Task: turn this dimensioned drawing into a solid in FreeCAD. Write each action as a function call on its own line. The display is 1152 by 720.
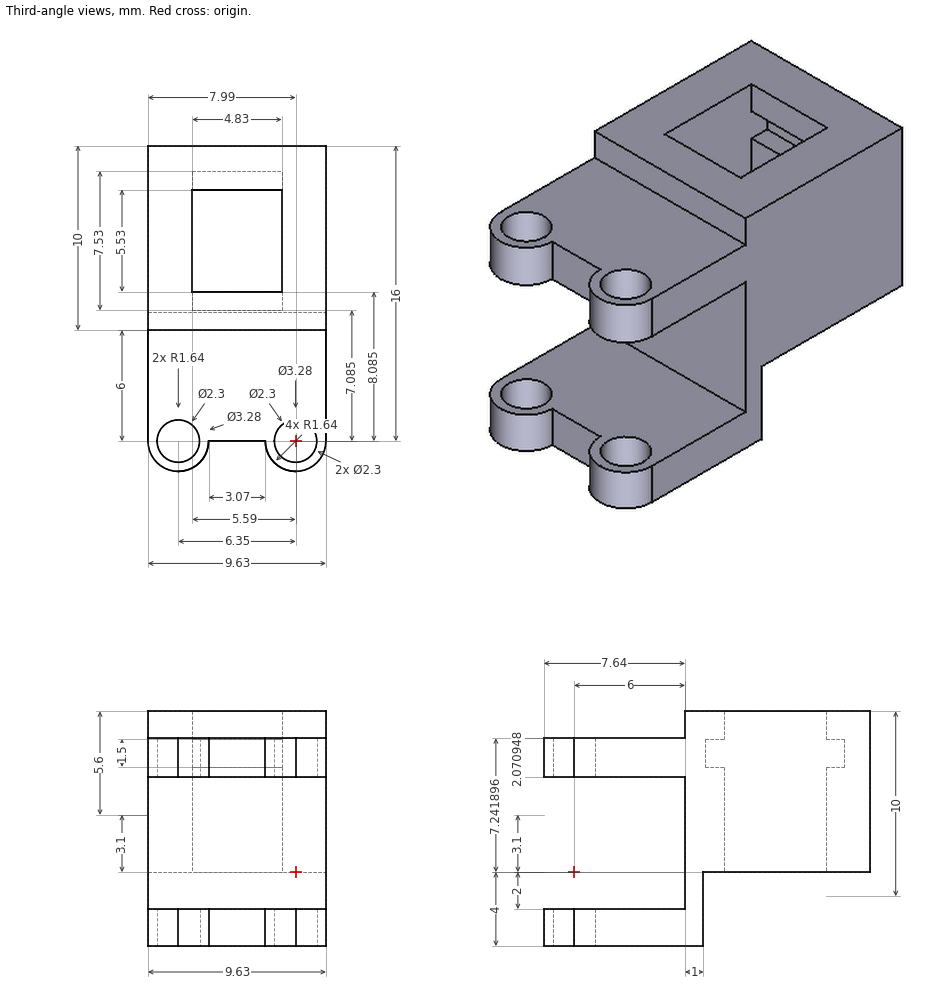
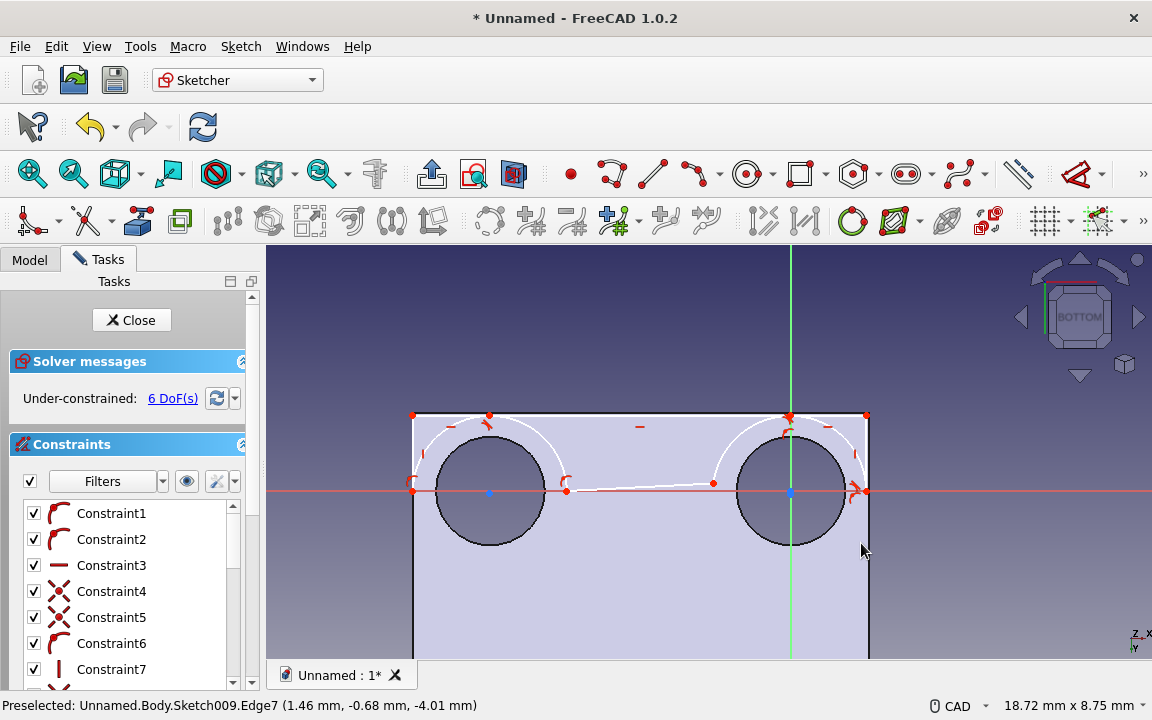
click(413, 438)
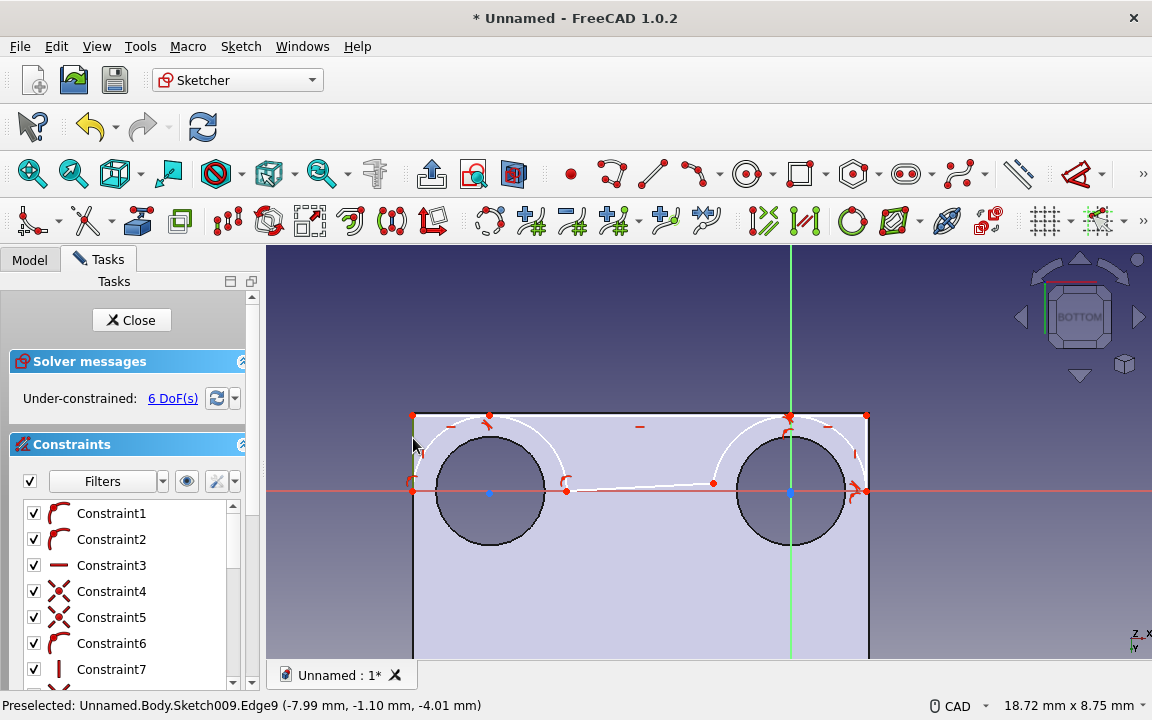
scroll(422, 457, up, 3)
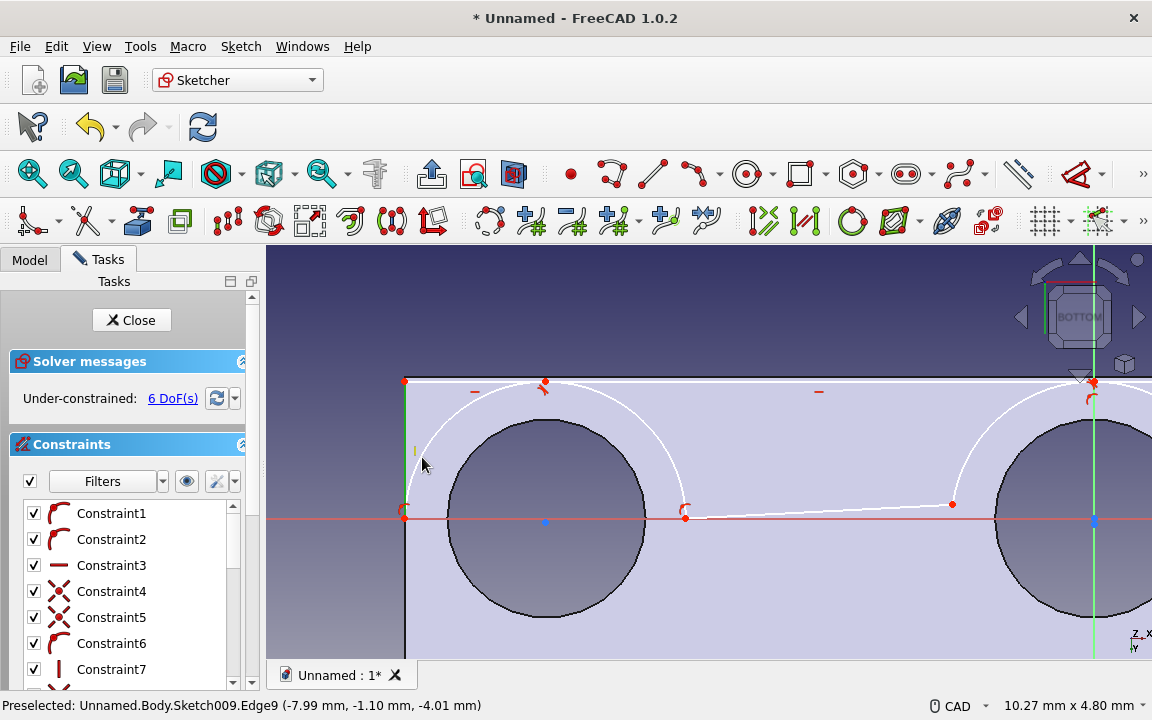
click(421, 456)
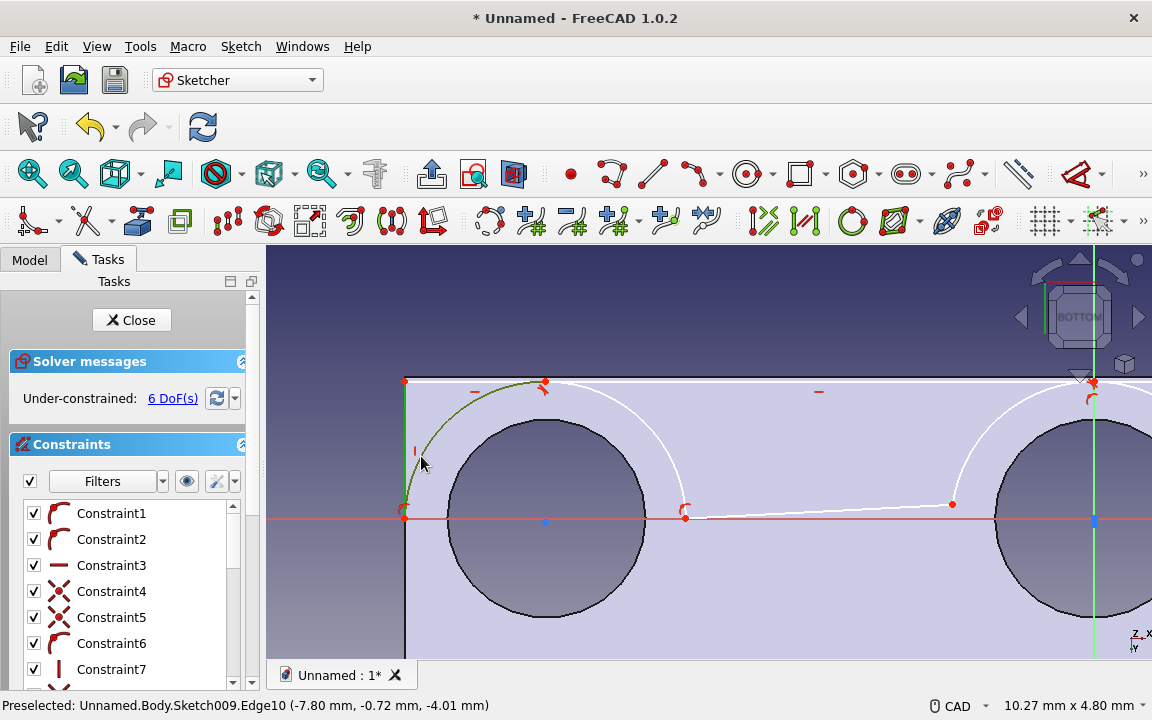
key(t)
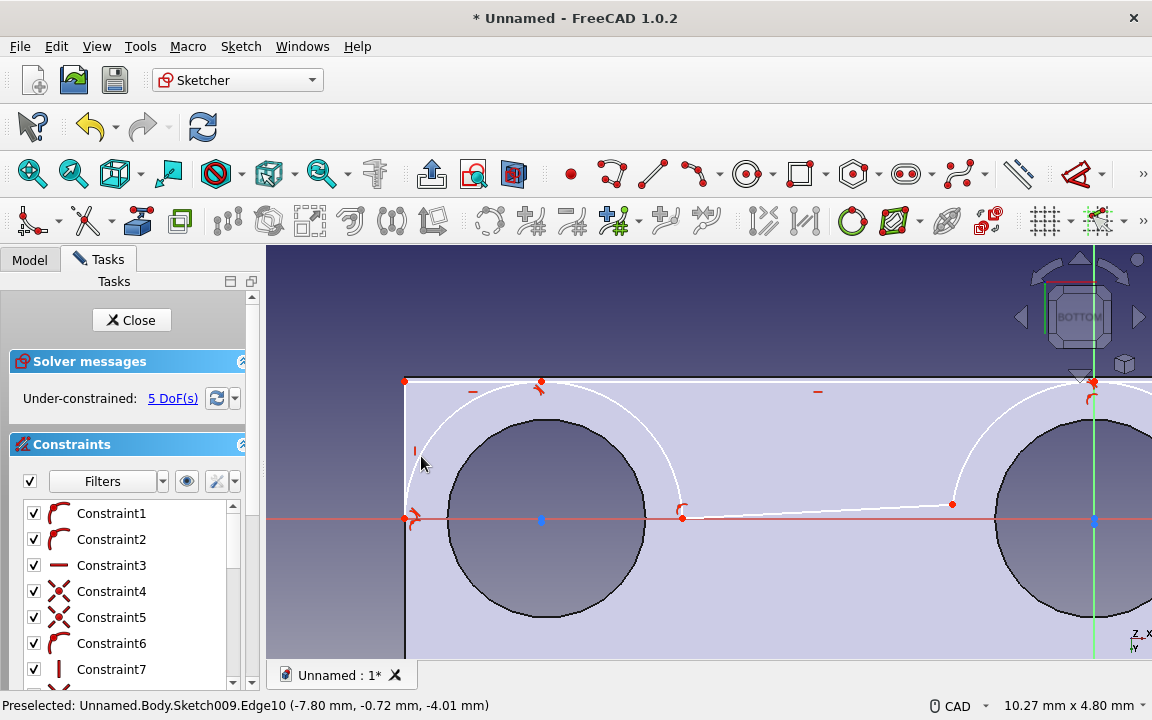
scroll(872, 509, up, 2)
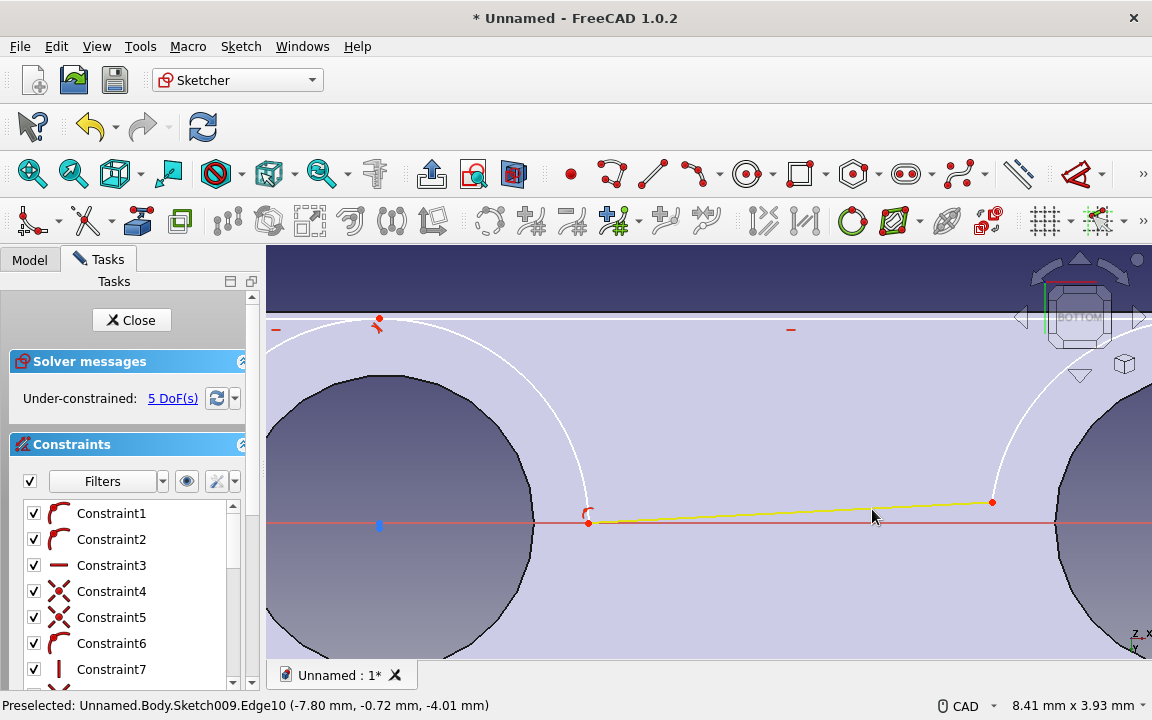
click(871, 509)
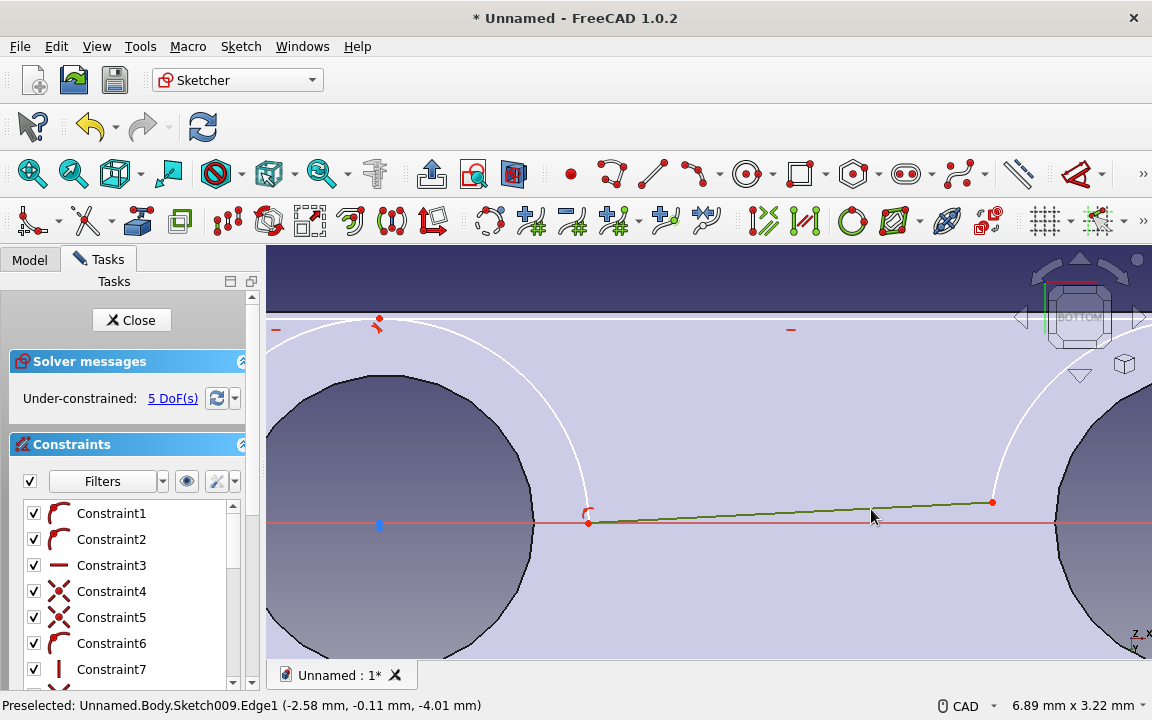
key(h)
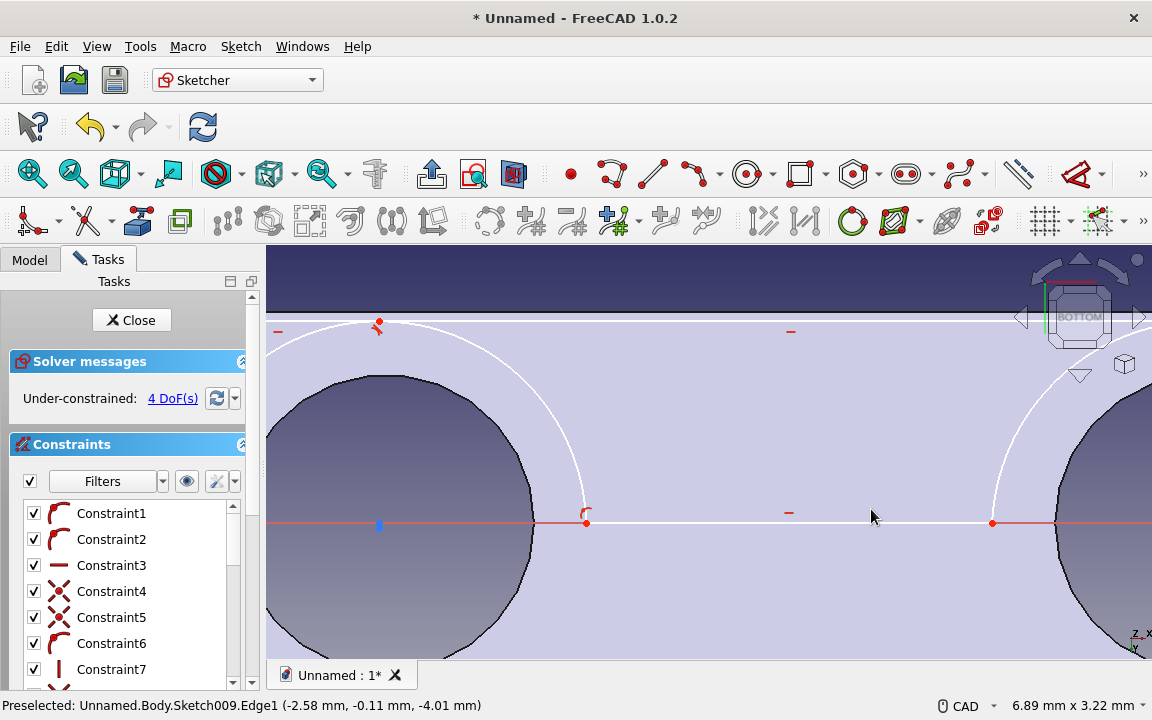
scroll(551, 472, down, 5)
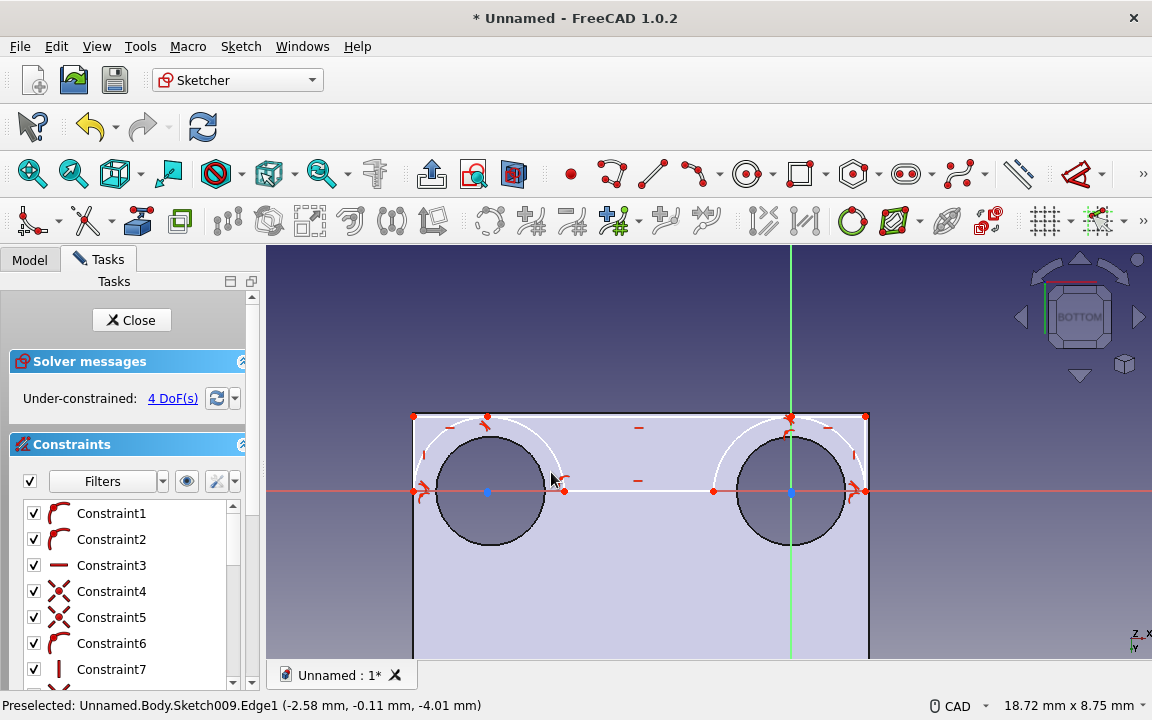
scroll(757, 425, up, 3)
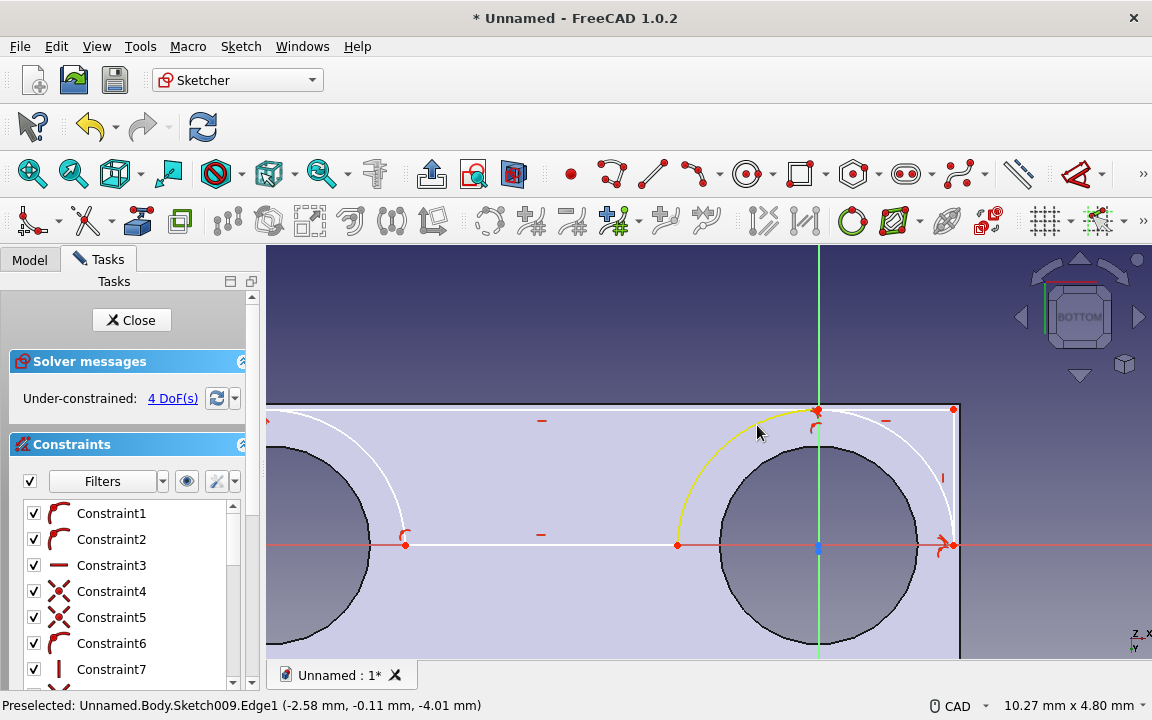
click(756, 424)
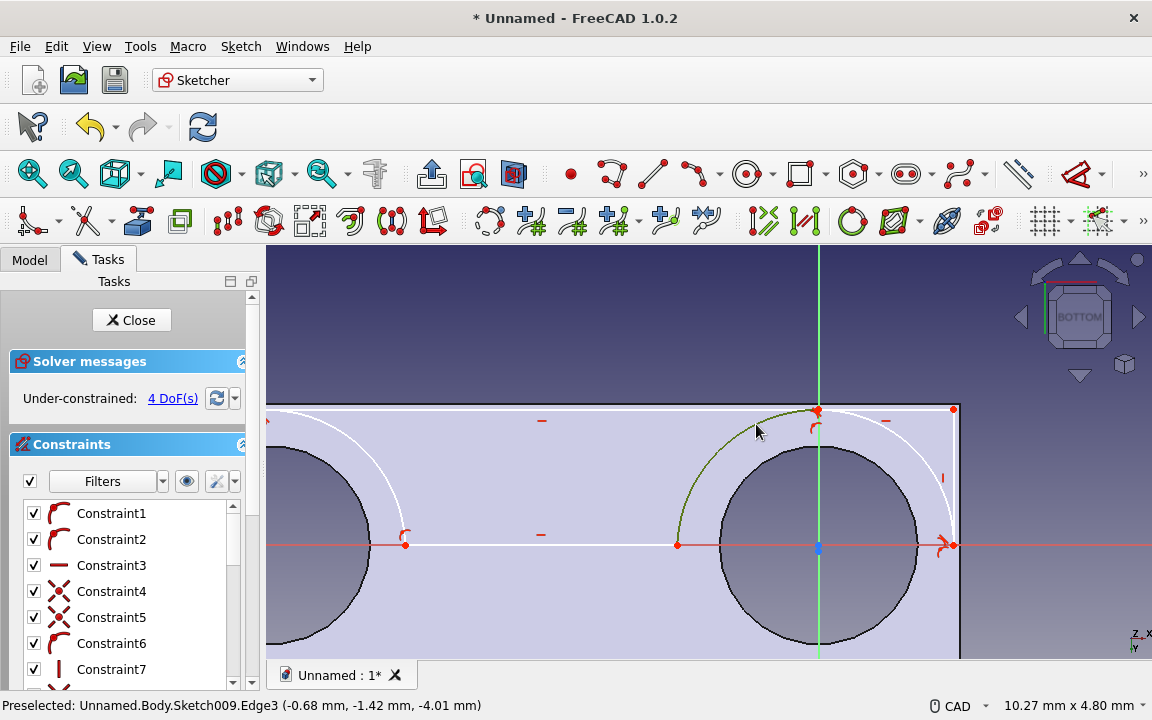
click(389, 483)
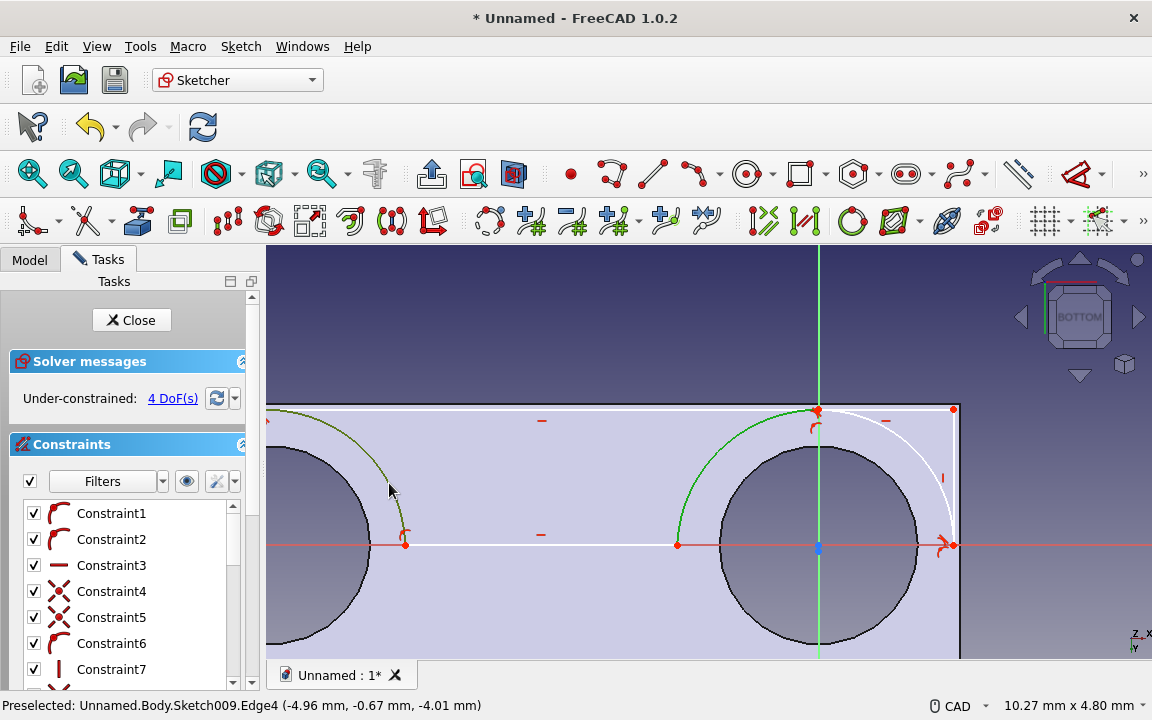
click(939, 484)